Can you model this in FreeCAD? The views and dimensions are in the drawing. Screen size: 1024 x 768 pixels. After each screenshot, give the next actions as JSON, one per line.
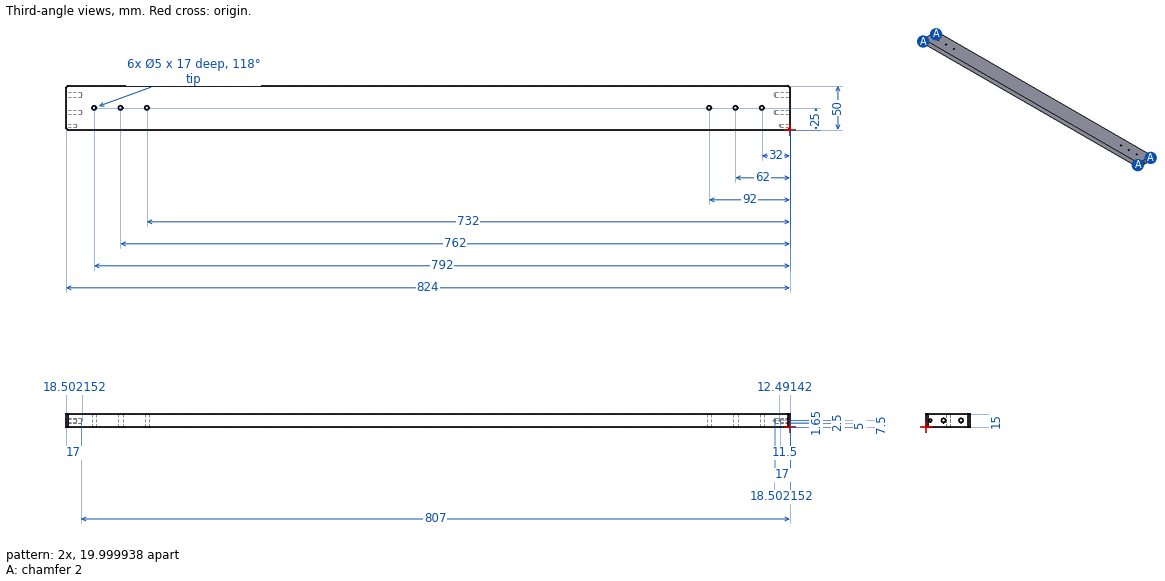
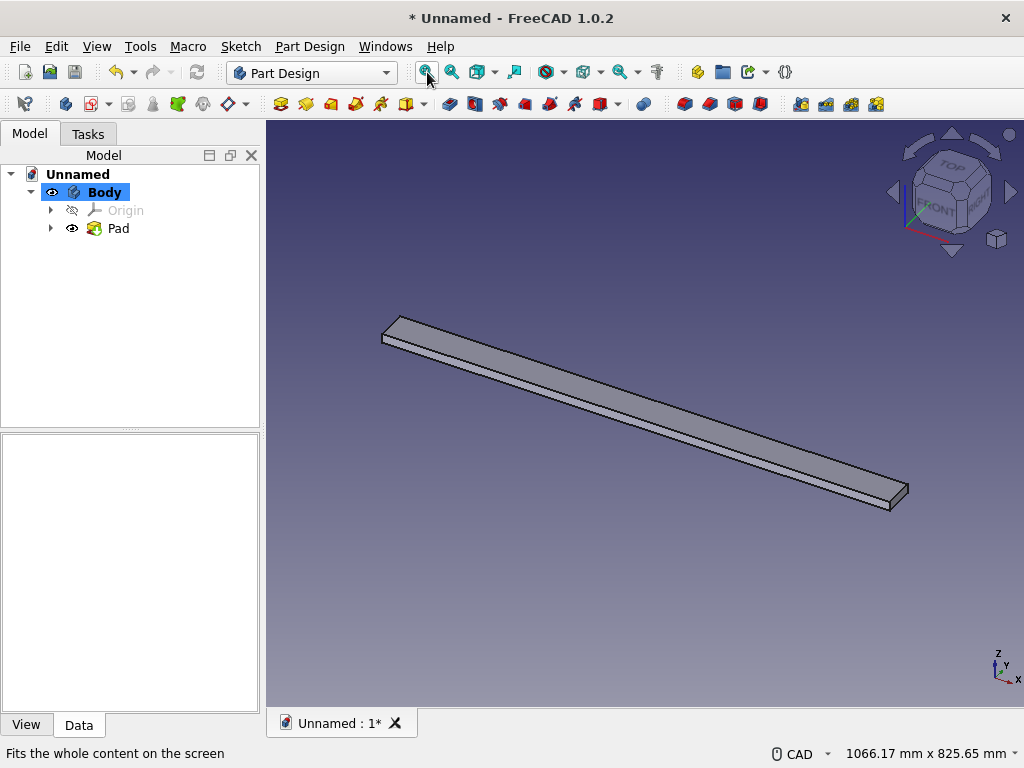
{"action": "left_click", "coordinate": [51, 210]}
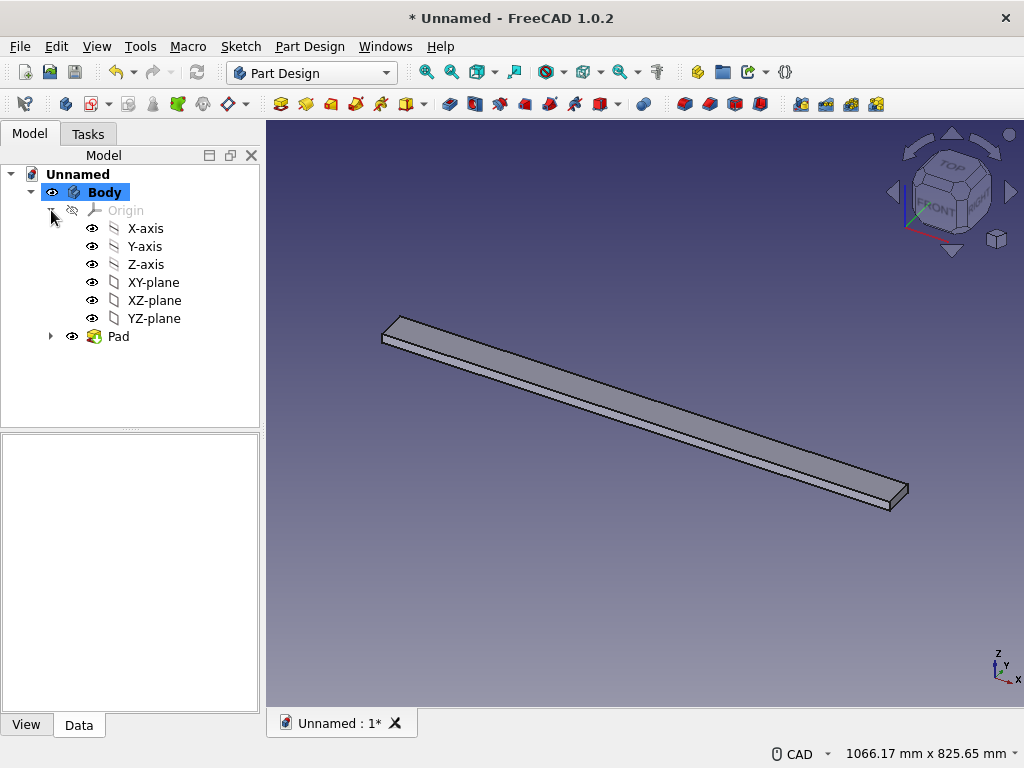
{"action": "left_click", "coordinate": [137, 300]}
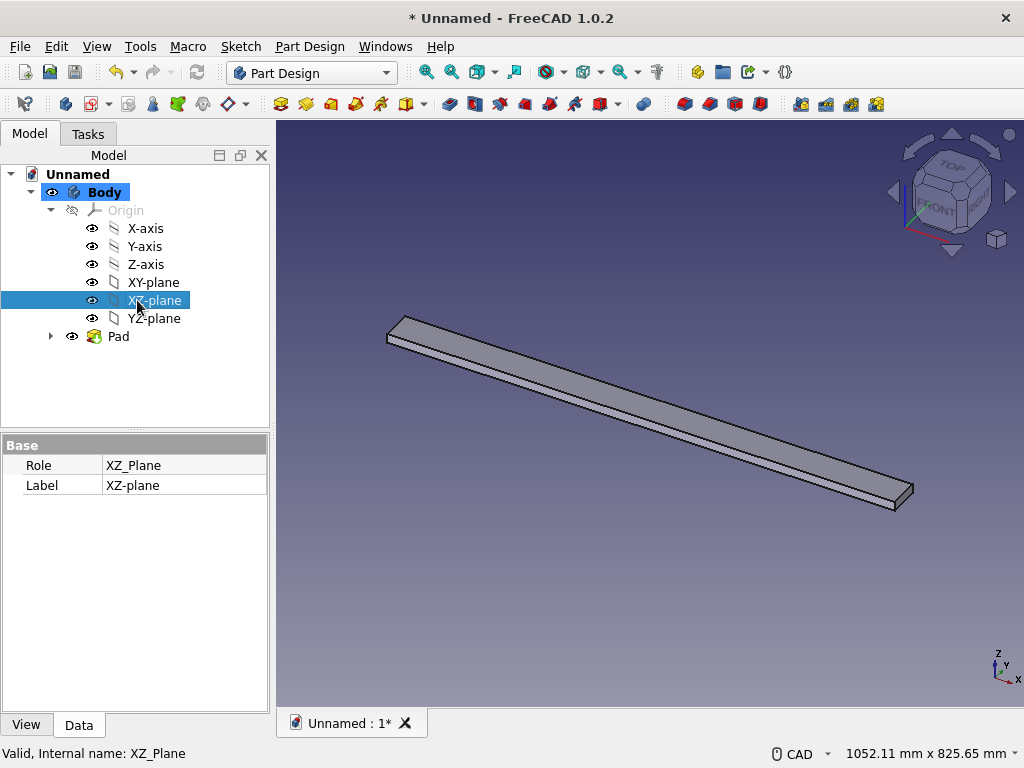
{"action": "left_click", "coordinate": [228, 104]}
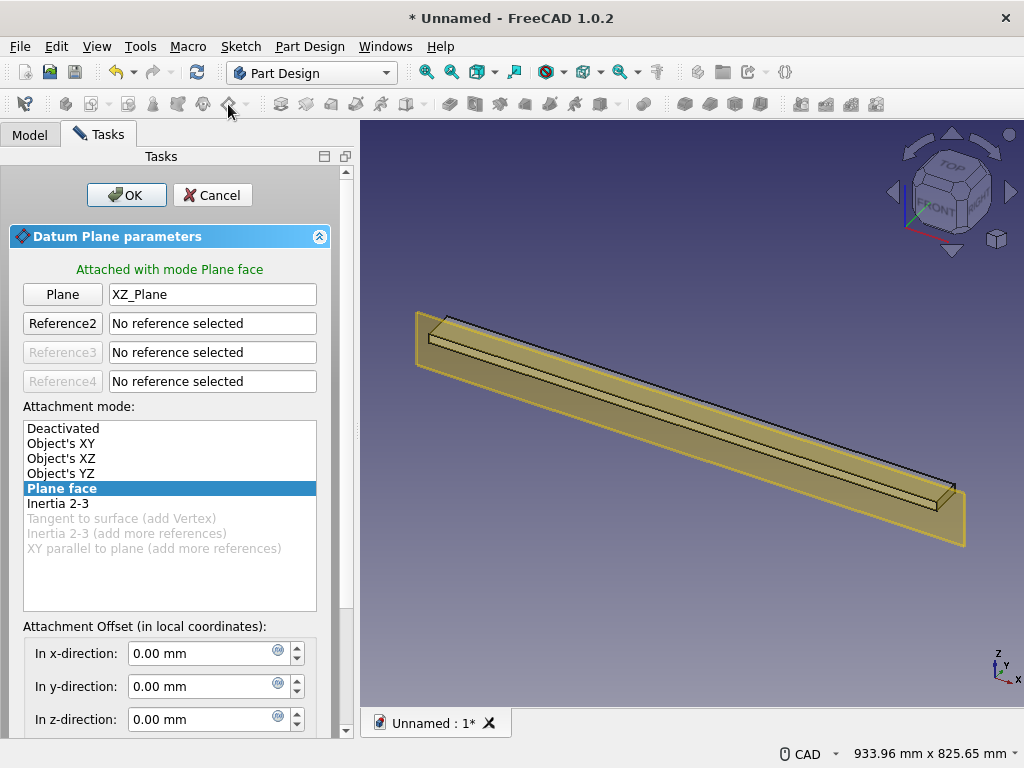
{"action": "triple_click", "coordinate": [210, 720]}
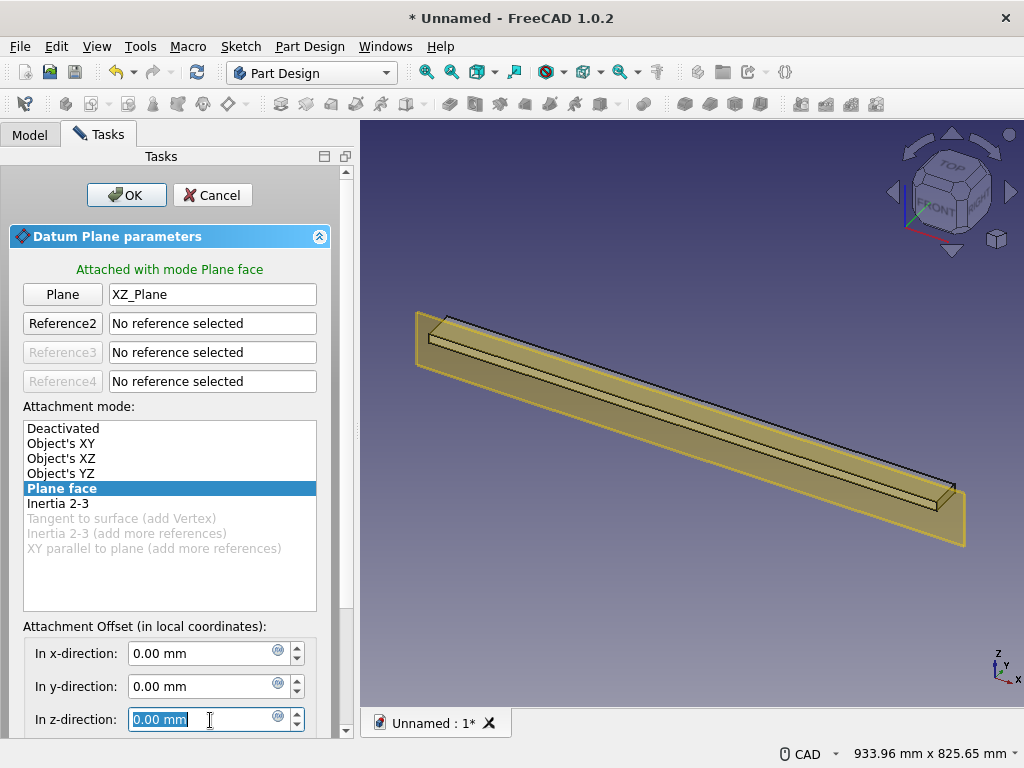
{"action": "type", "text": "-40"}
{"action": "key", "text": "Tab"}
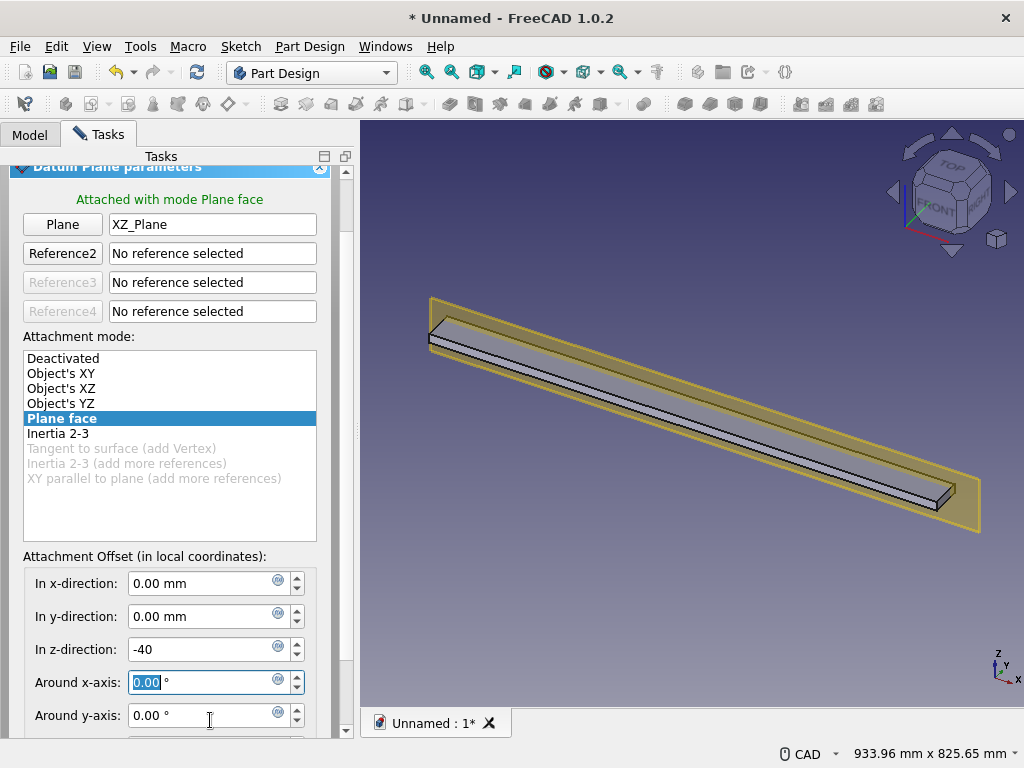
{"action": "scroll", "coordinate": [346, 452], "scroll_direction": "up", "scroll_amount": 2}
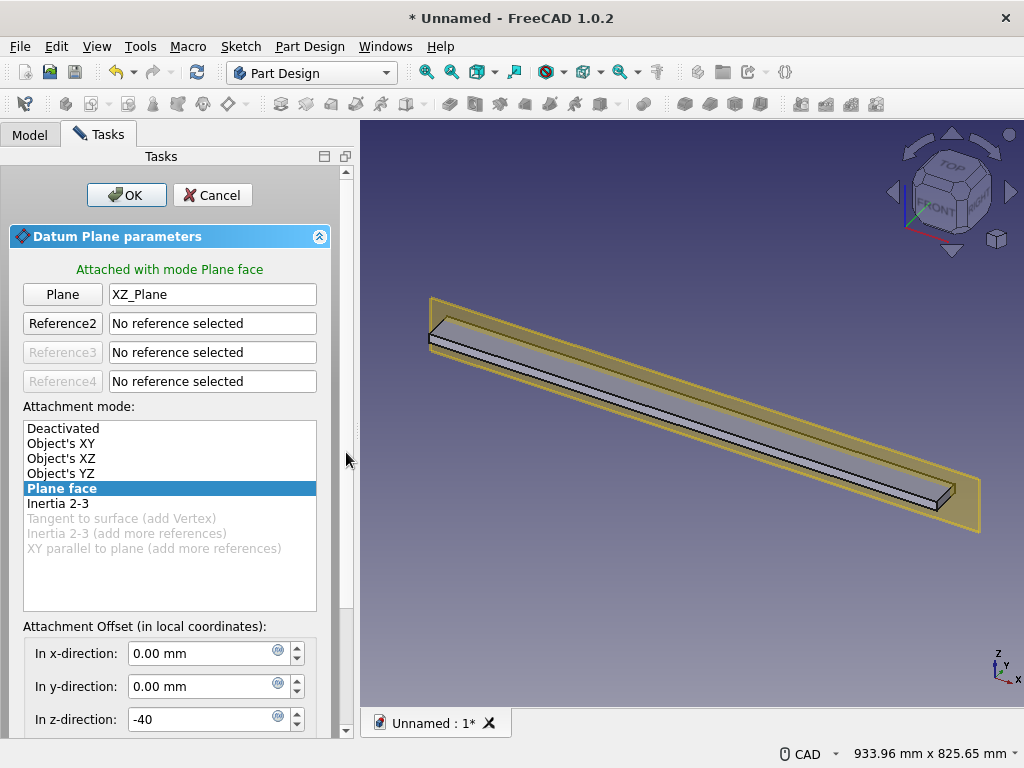
{"action": "left_click", "coordinate": [127, 195]}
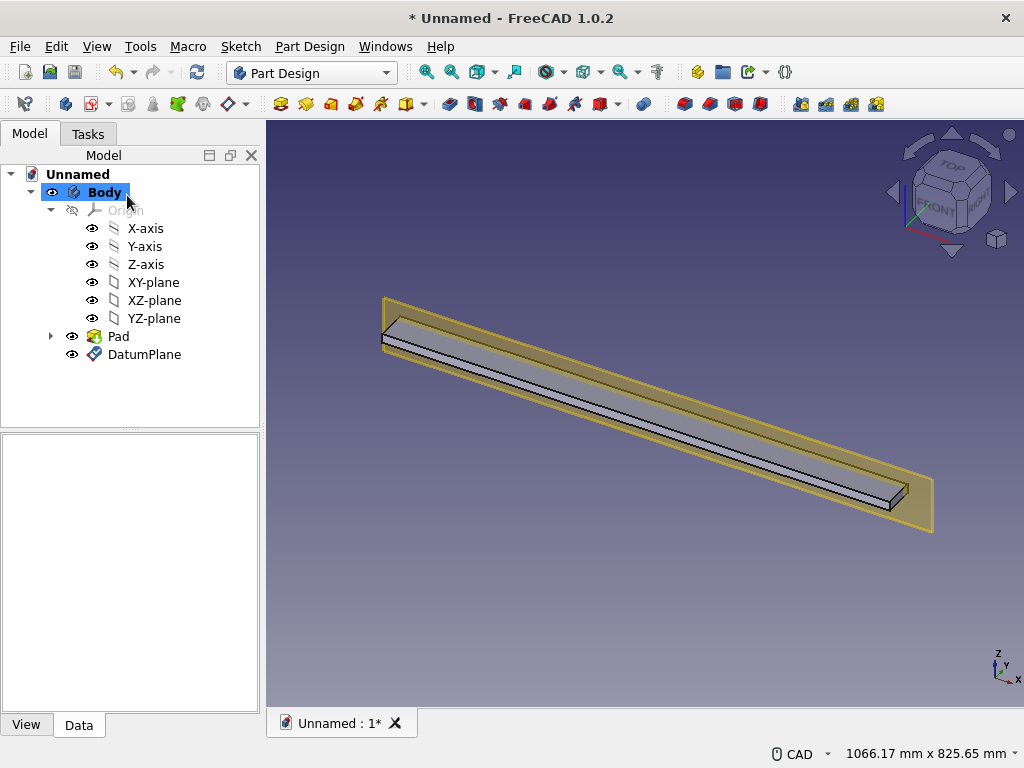
{"action": "left_click", "coordinate": [117, 354]}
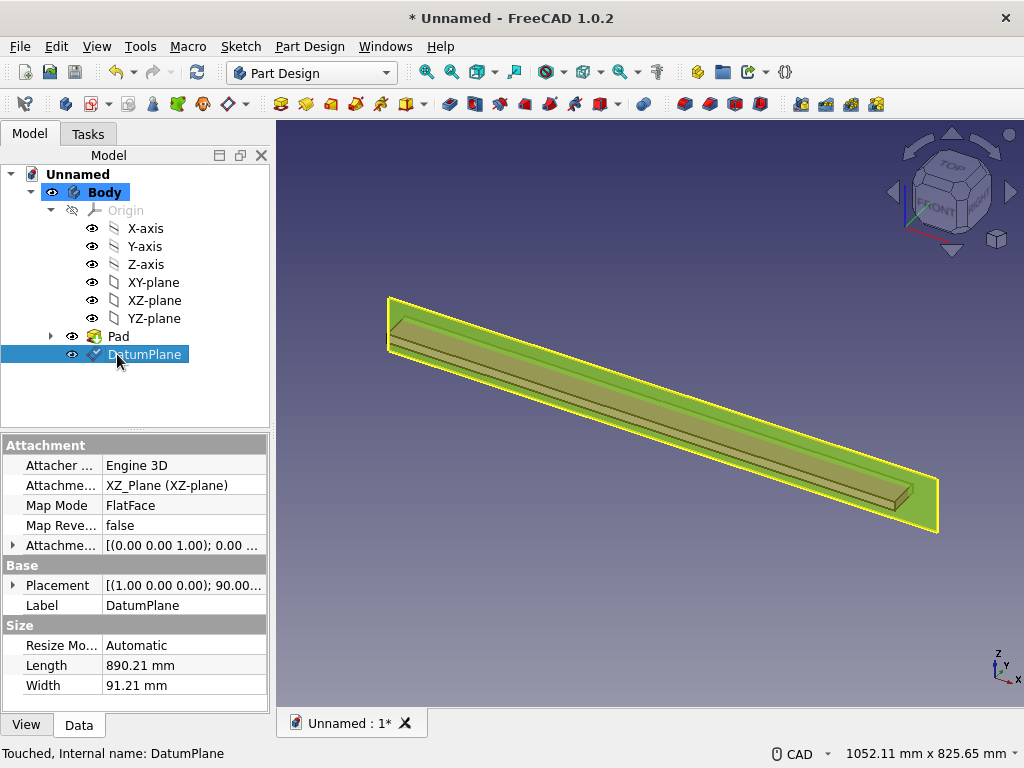
{"action": "left_click", "coordinate": [90, 104]}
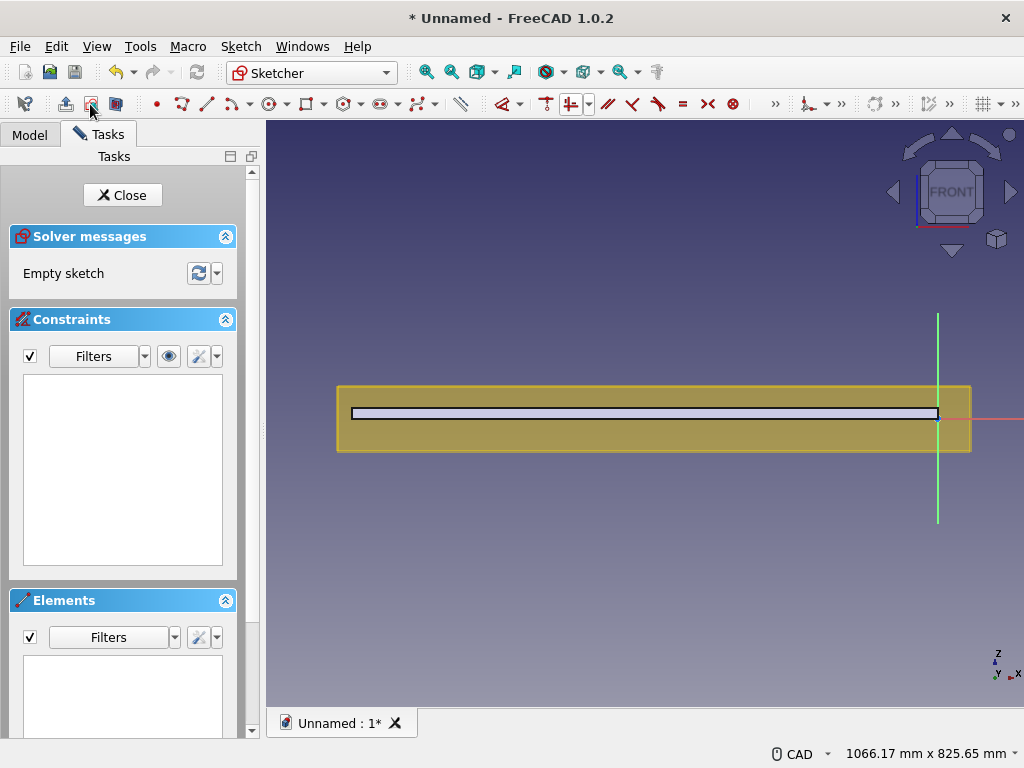
{"action": "left_click", "coordinate": [116, 104]}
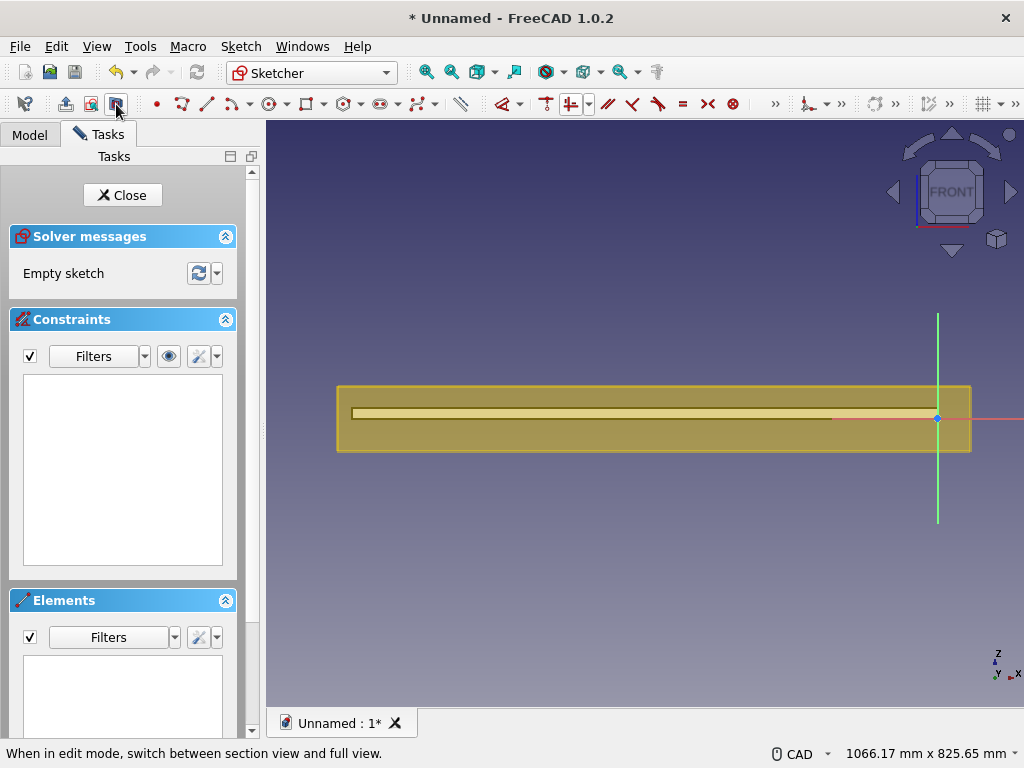
{"action": "scroll", "coordinate": [576, 414], "scroll_direction": "down", "scroll_amount": 5}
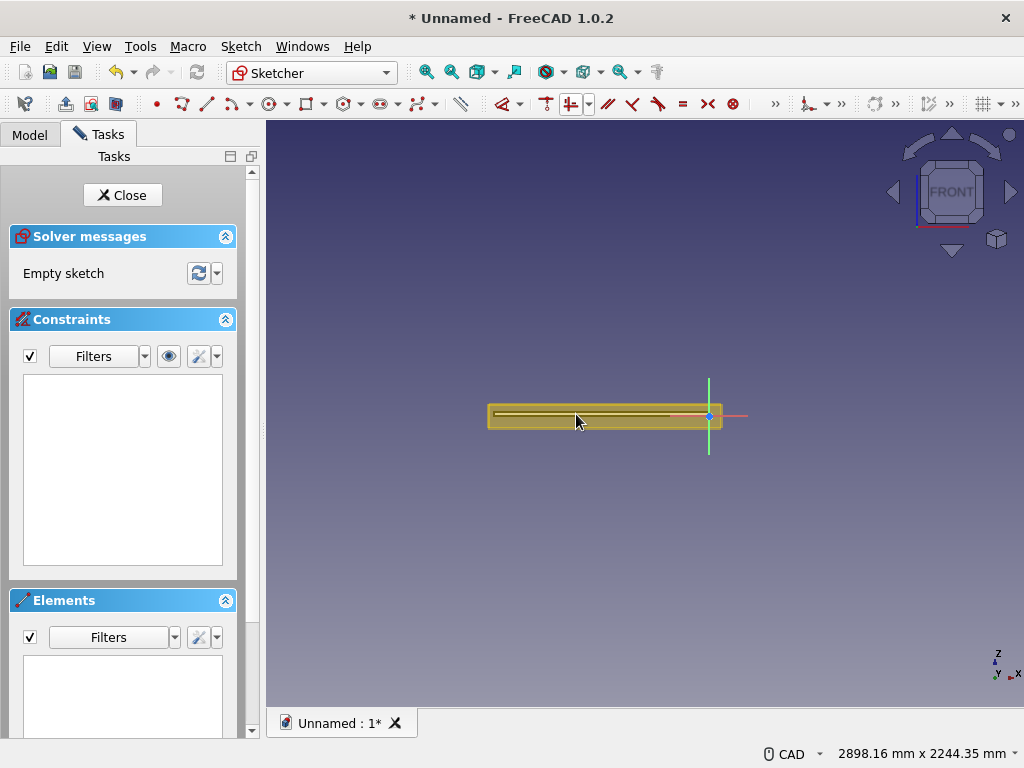
{"action": "scroll", "coordinate": [713, 415], "scroll_direction": "up", "scroll_amount": 15}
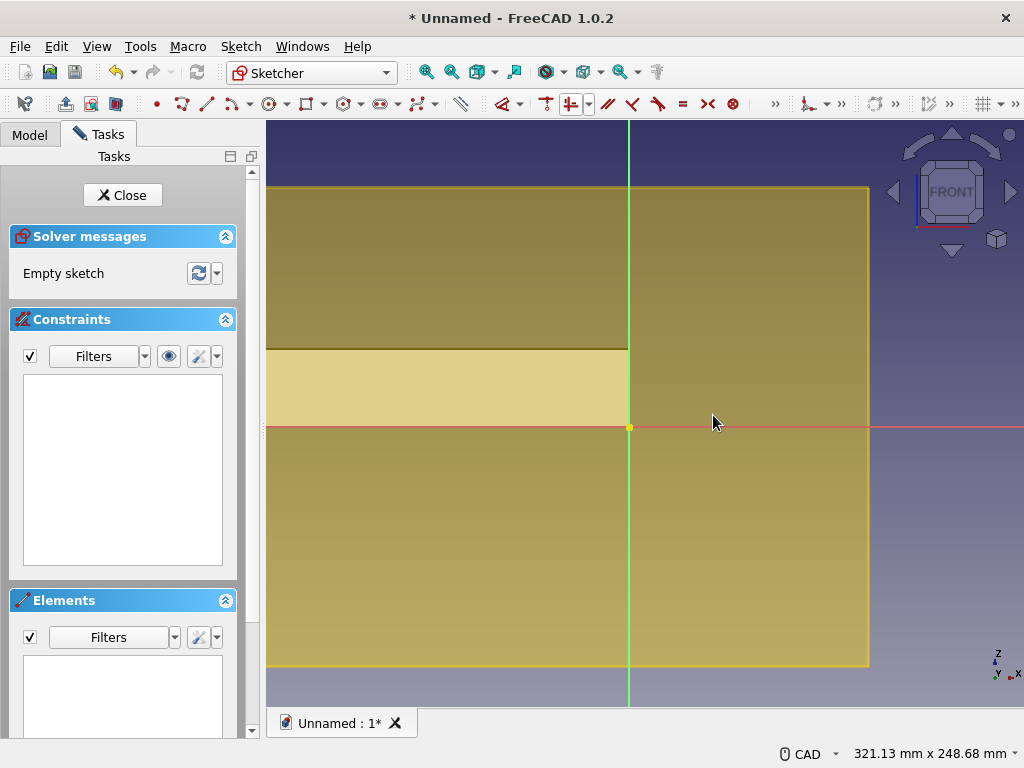
{"action": "scroll", "coordinate": [553, 404], "scroll_direction": "up", "scroll_amount": 5}